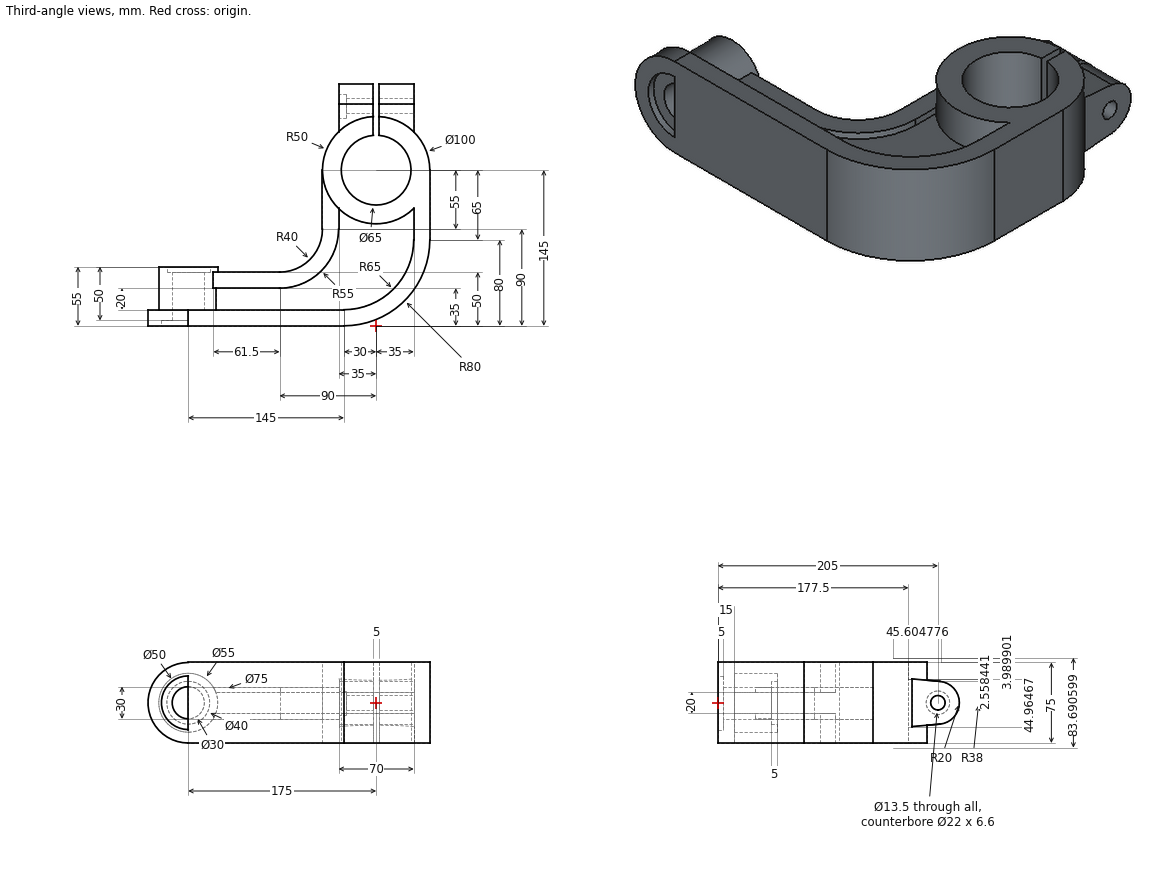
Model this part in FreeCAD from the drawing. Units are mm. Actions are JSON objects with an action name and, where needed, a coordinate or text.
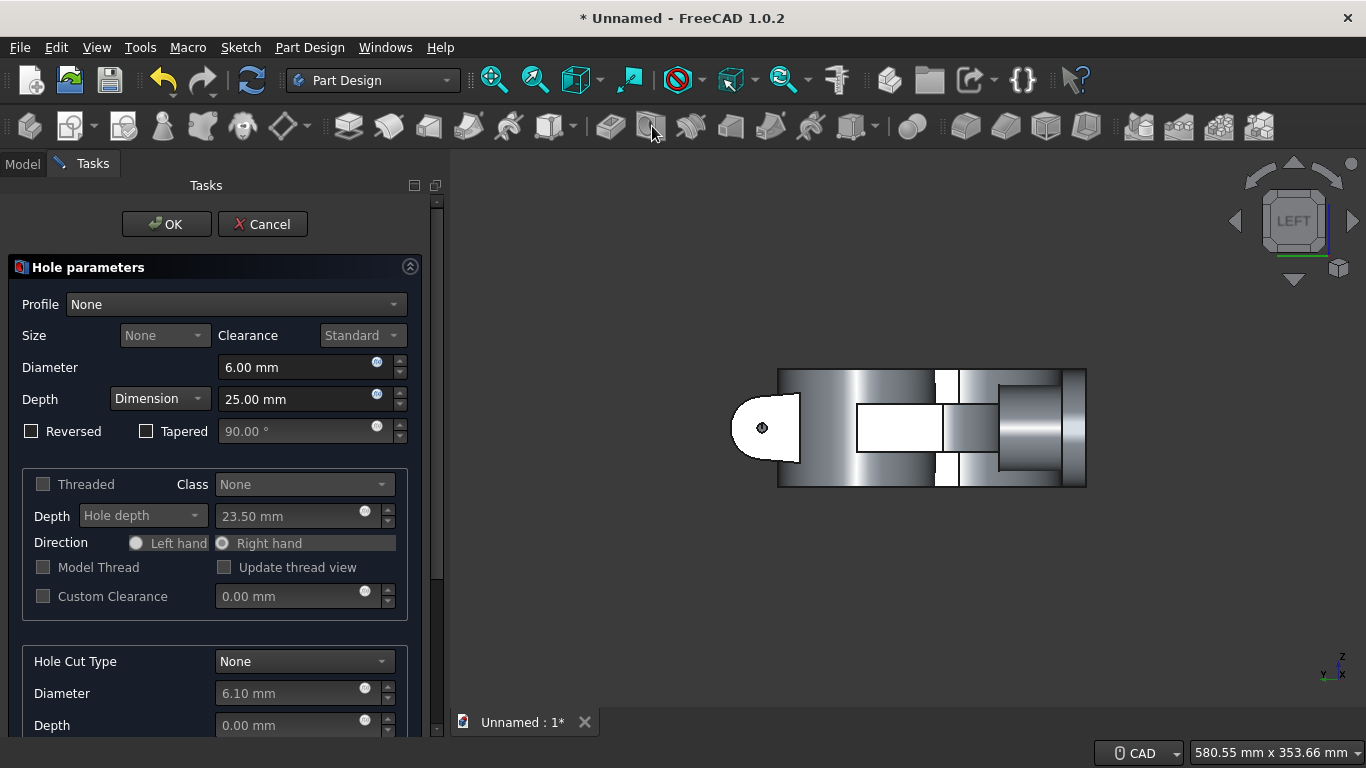
{"action": "triple_click", "coordinate": [305, 367]}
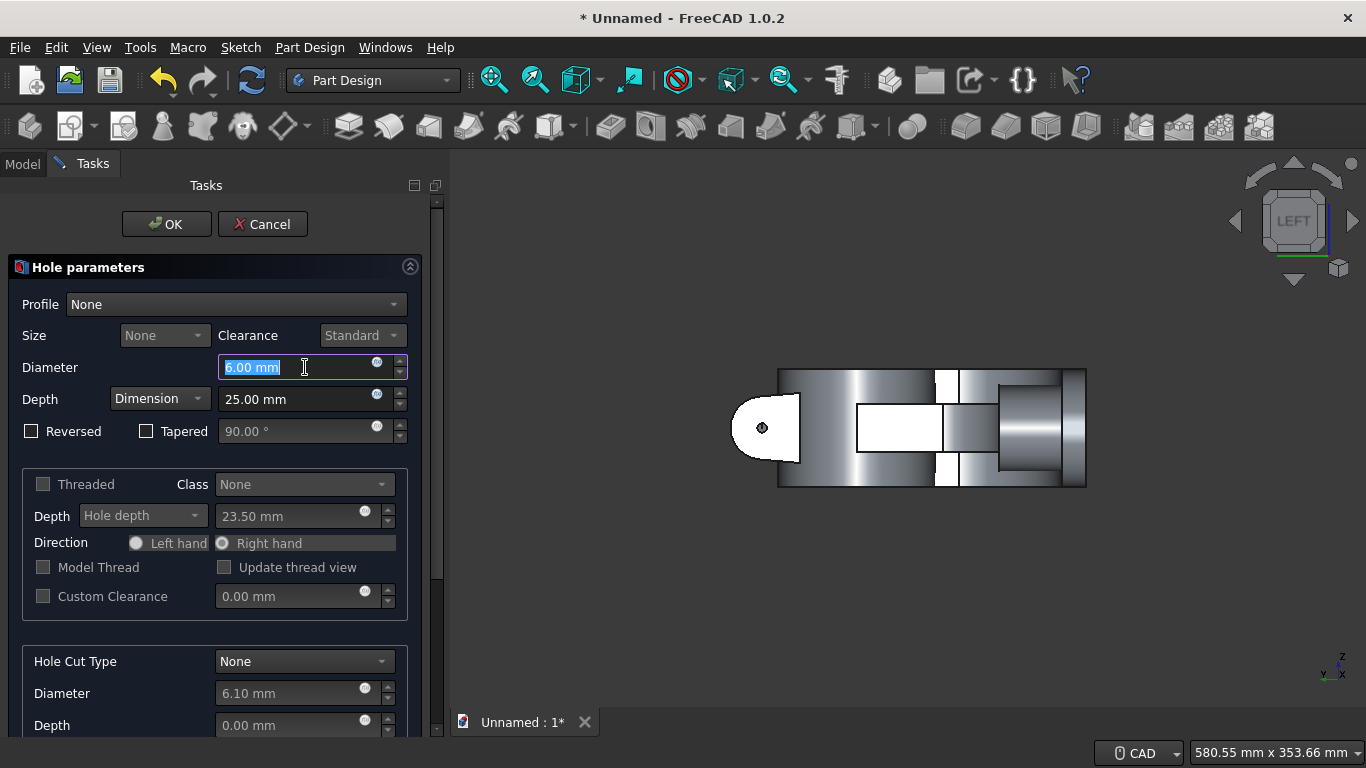
{"action": "type", "text": "13.5"}
{"action": "key", "text": "Tab"}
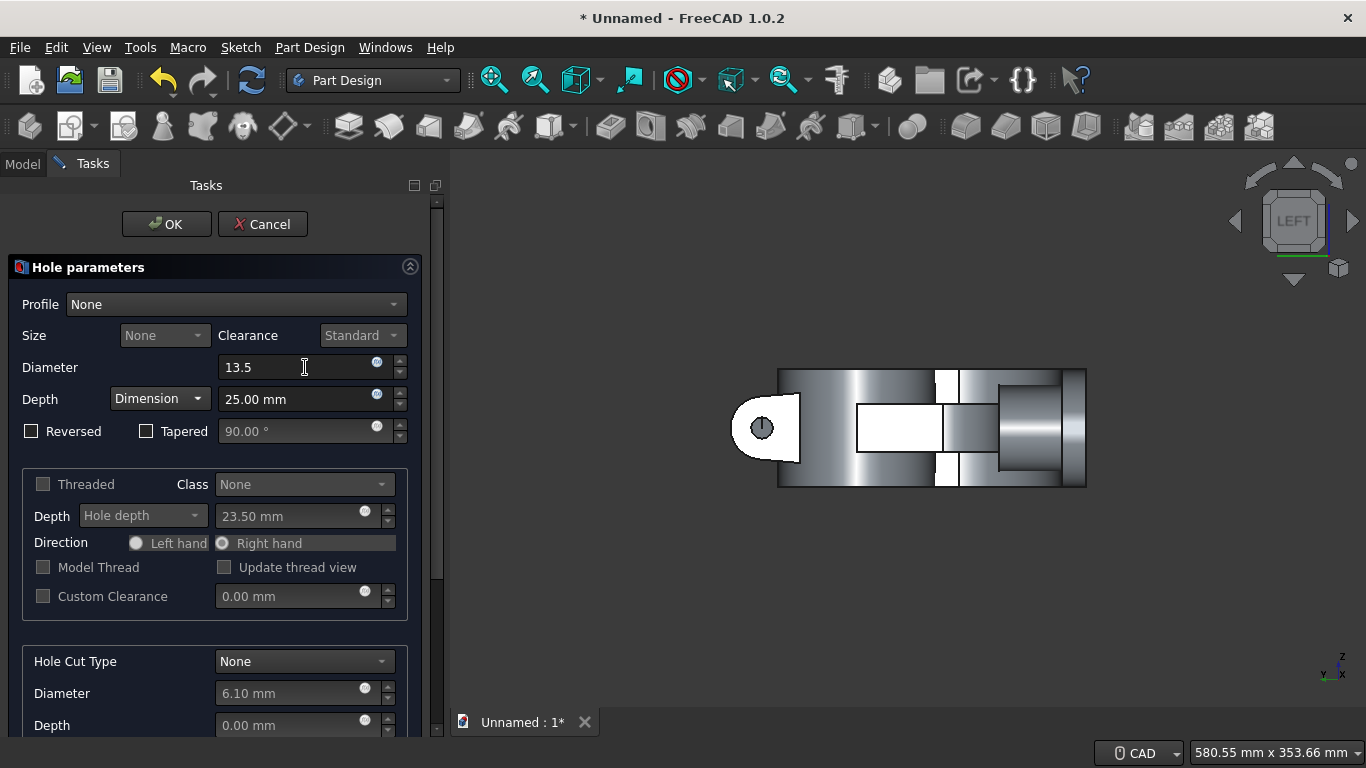
{"action": "left_click", "coordinate": [161, 398]}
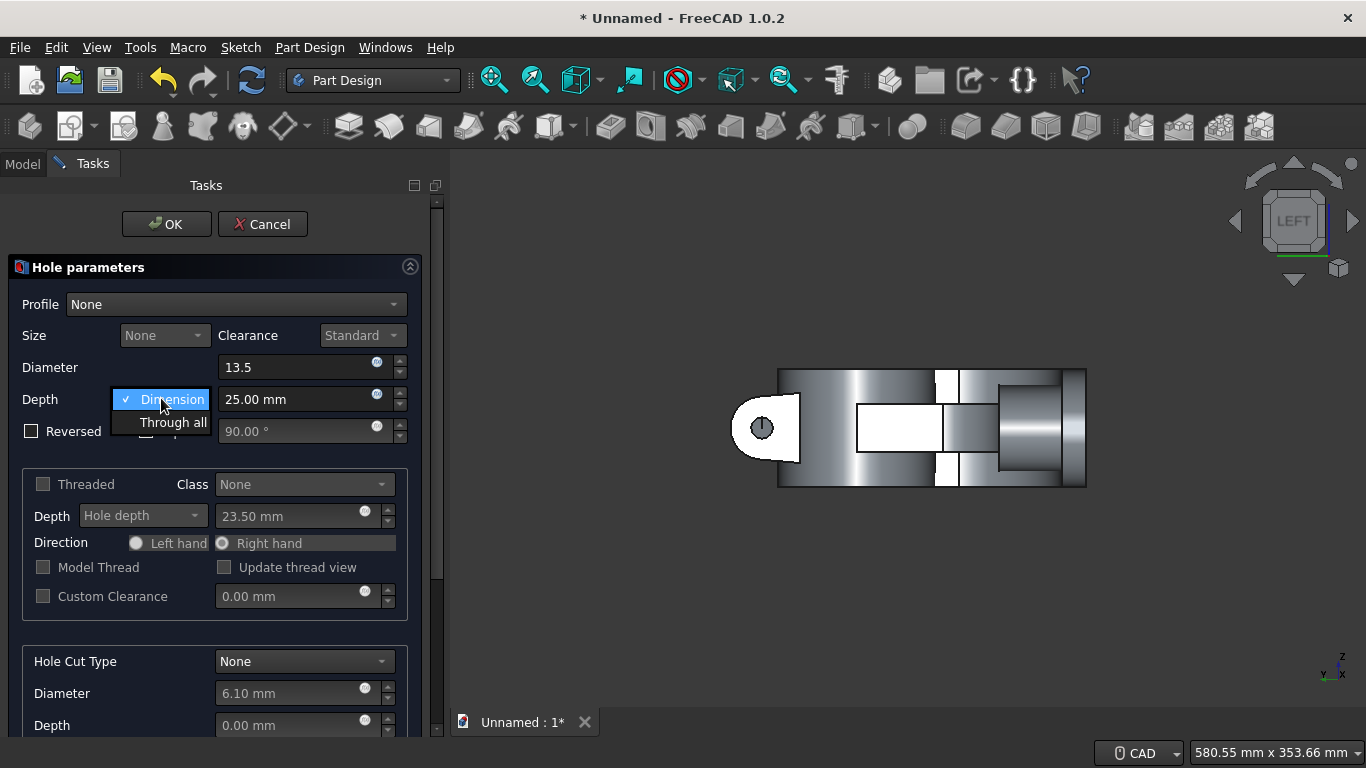
{"action": "left_click", "coordinate": [160, 422]}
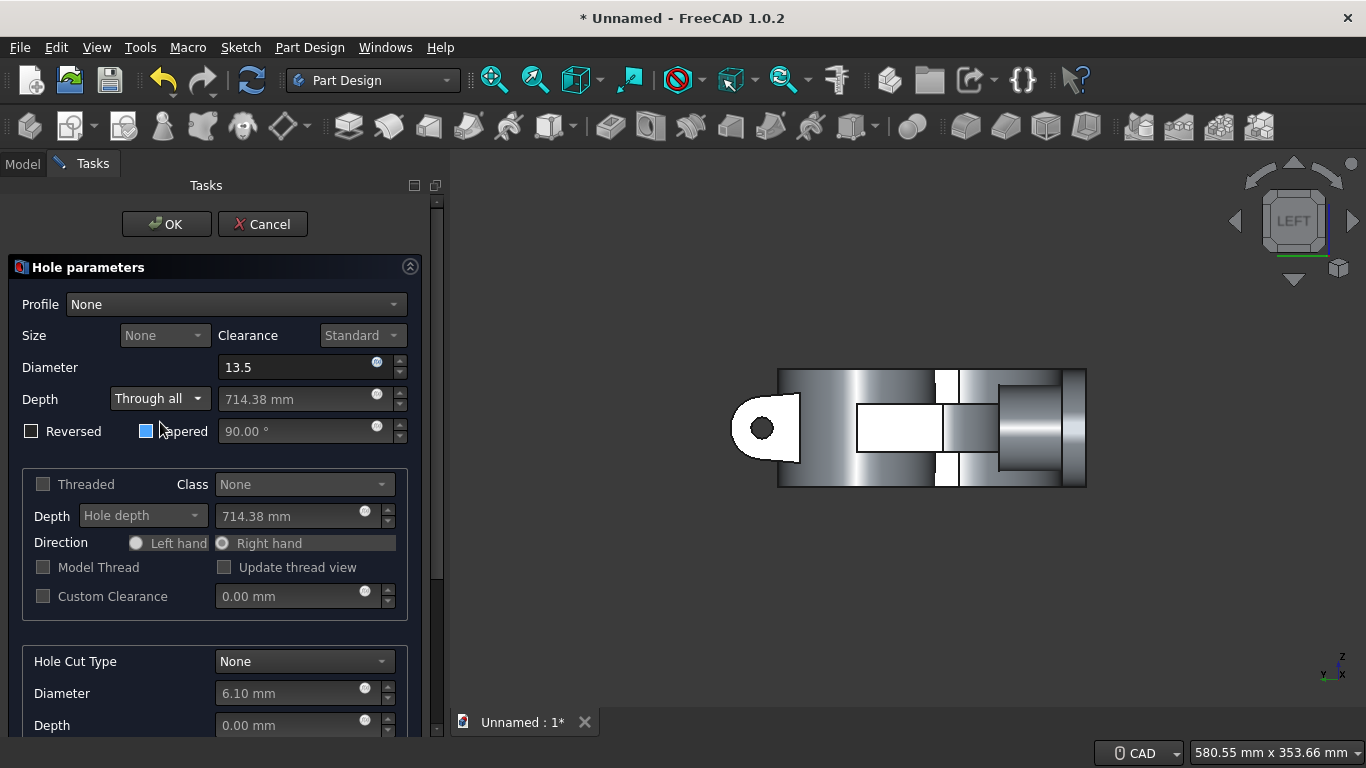
{"action": "left_click", "coordinate": [306, 662]}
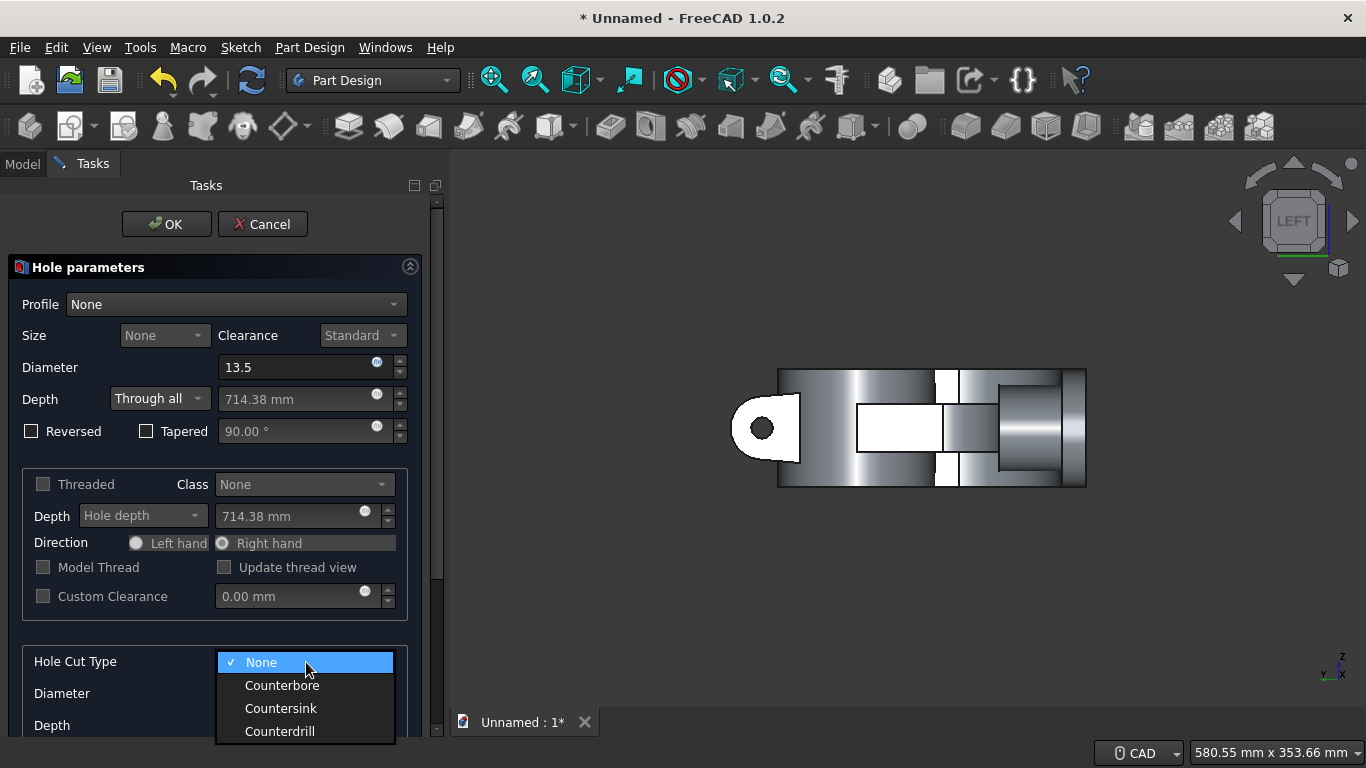
{"action": "left_click", "coordinate": [304, 686]}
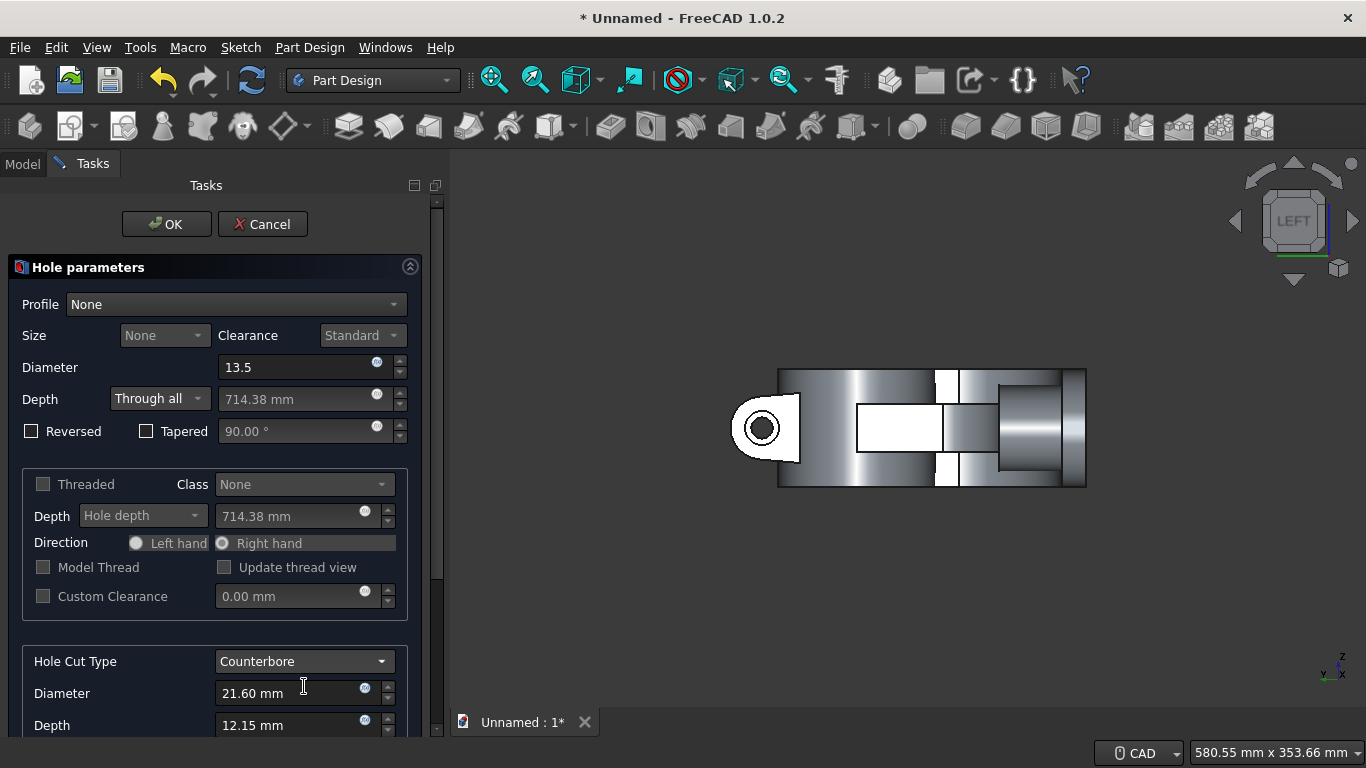
{"action": "triple_click", "coordinate": [298, 693]}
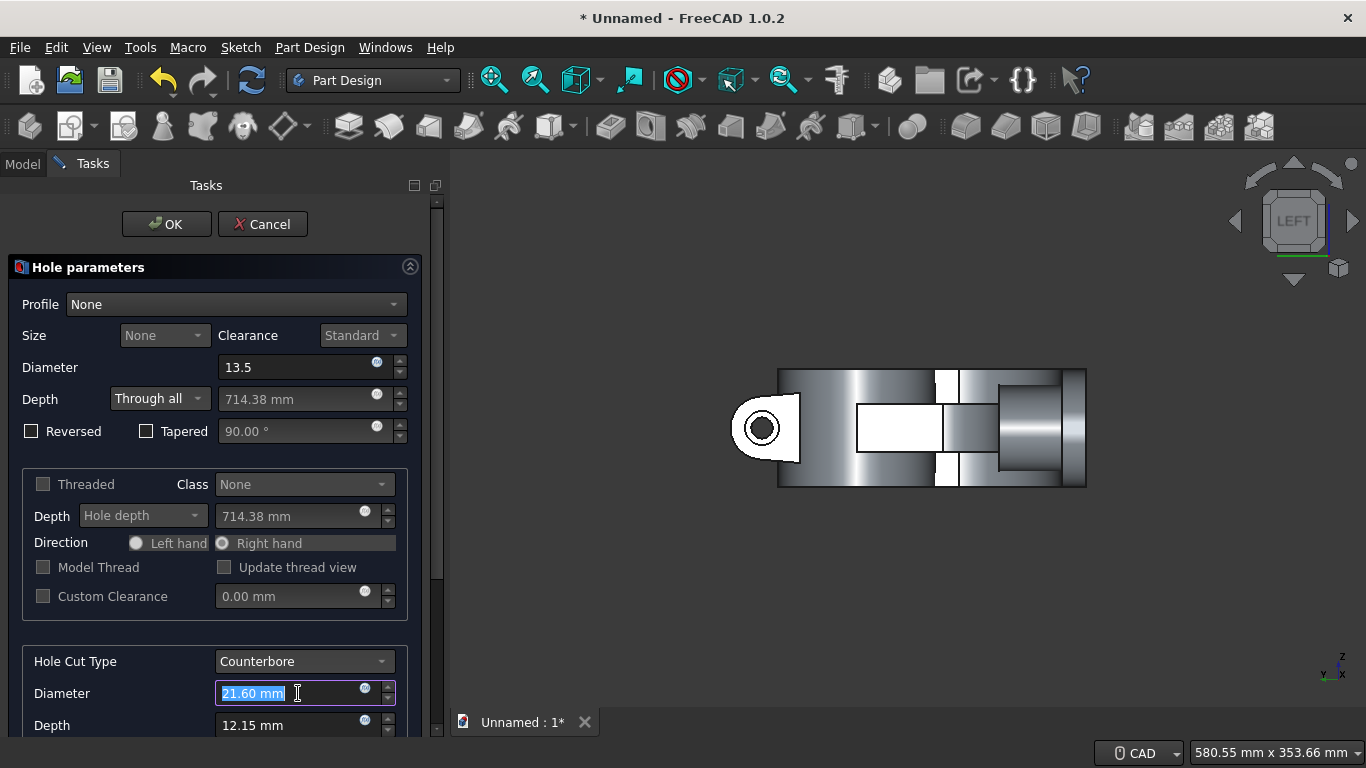
{"action": "type", "text": "22"}
{"action": "key", "text": "Tab"}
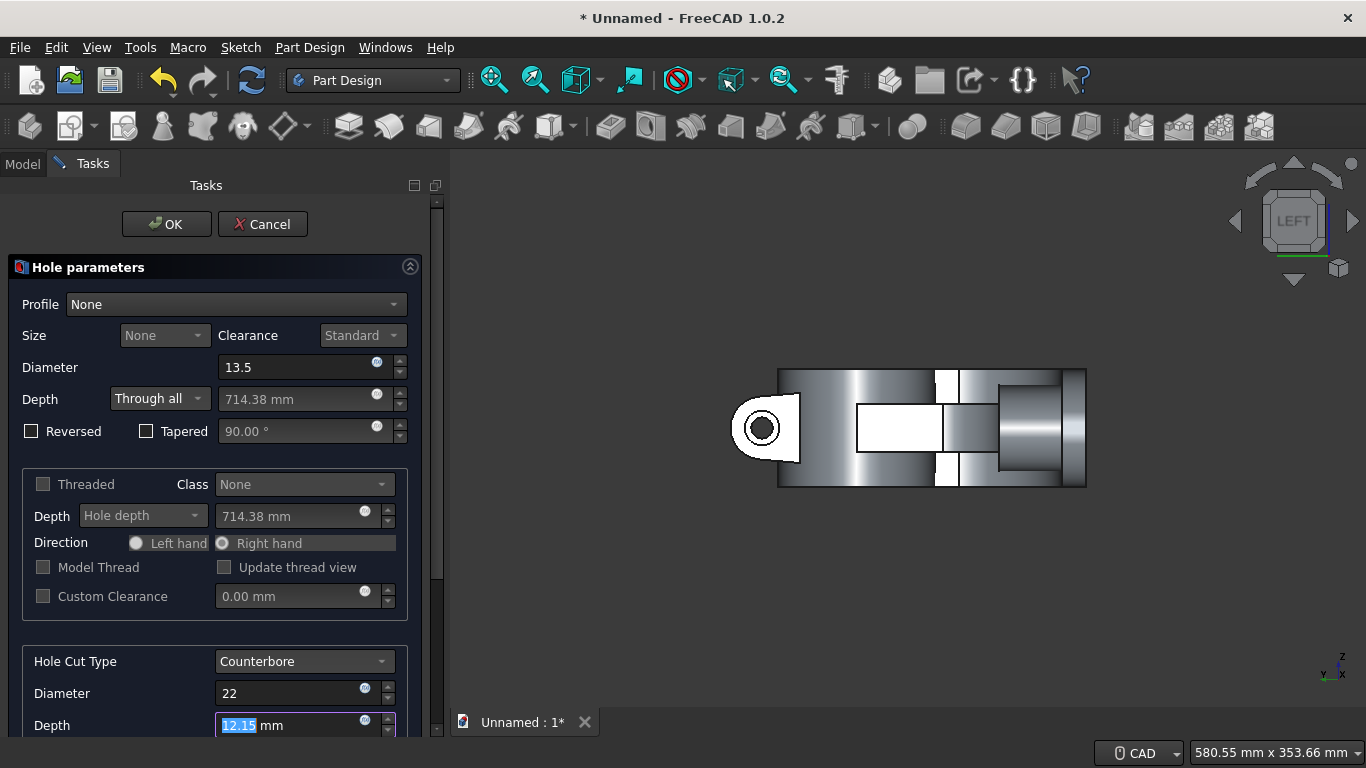
{"action": "scroll", "coordinate": [437, 466], "scroll_direction": "down", "scroll_amount": 2}